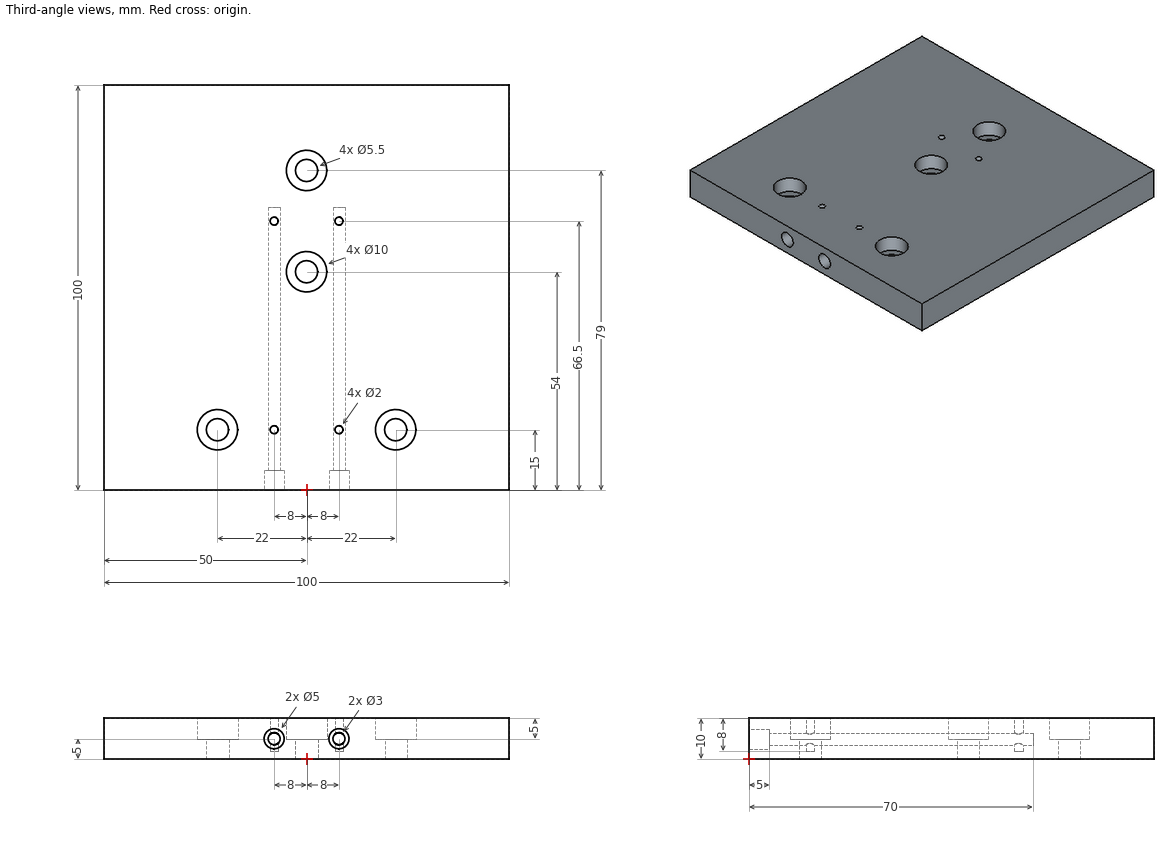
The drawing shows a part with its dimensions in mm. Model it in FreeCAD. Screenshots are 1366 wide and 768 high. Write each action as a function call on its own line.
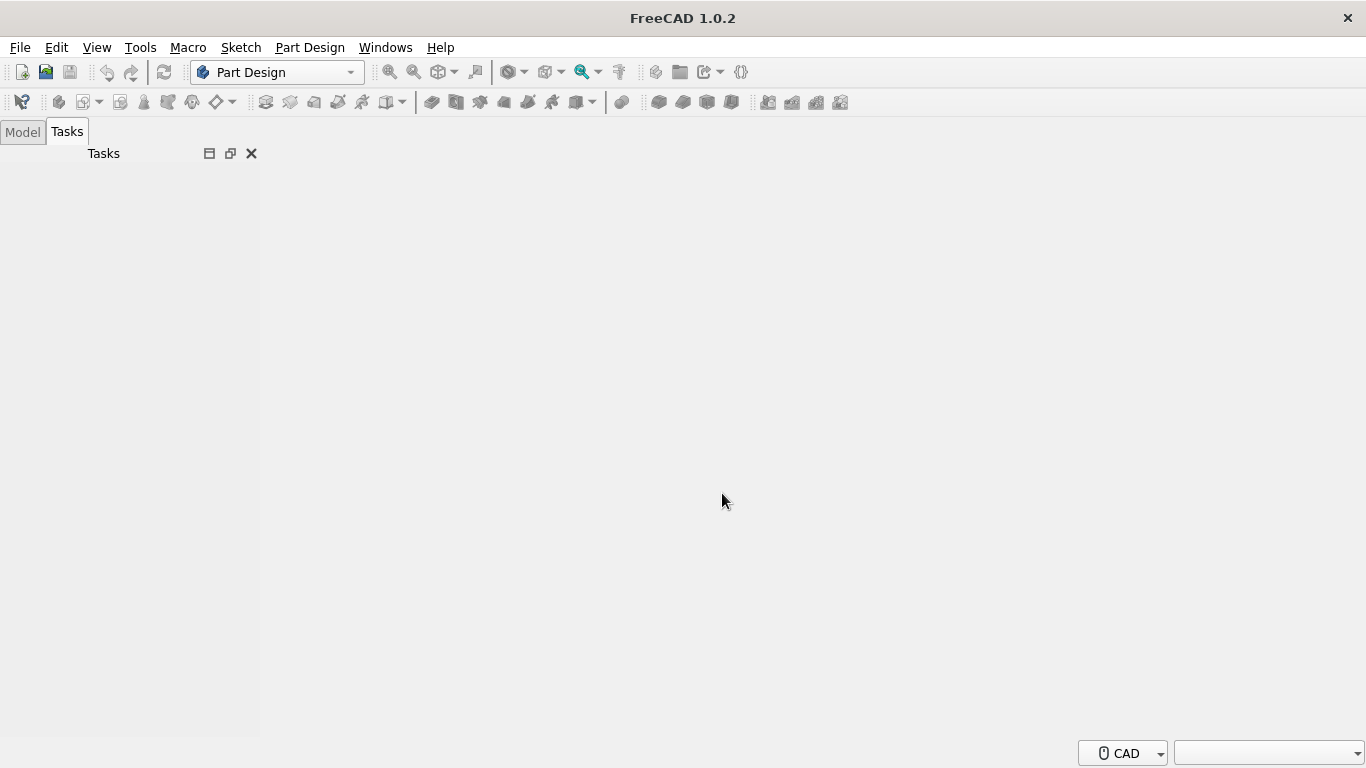
click(22, 72)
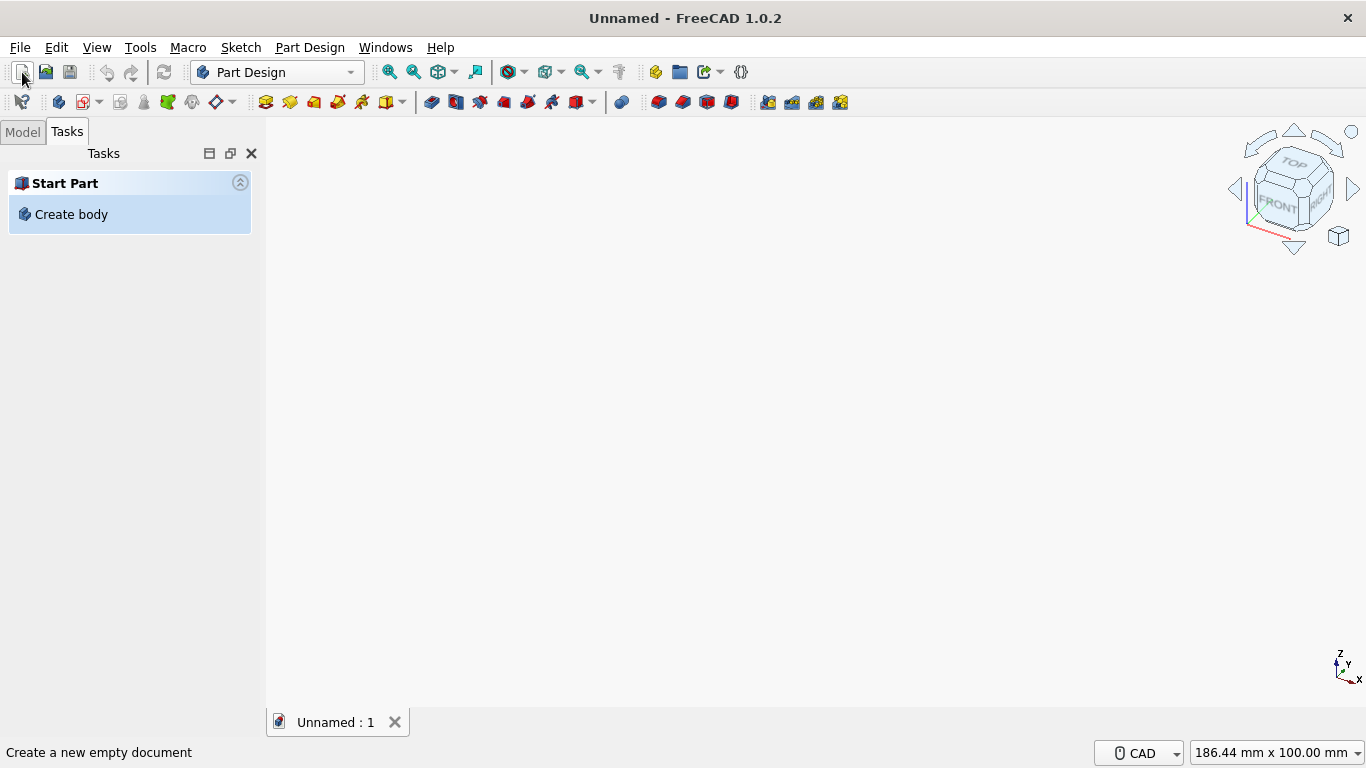
click(84, 102)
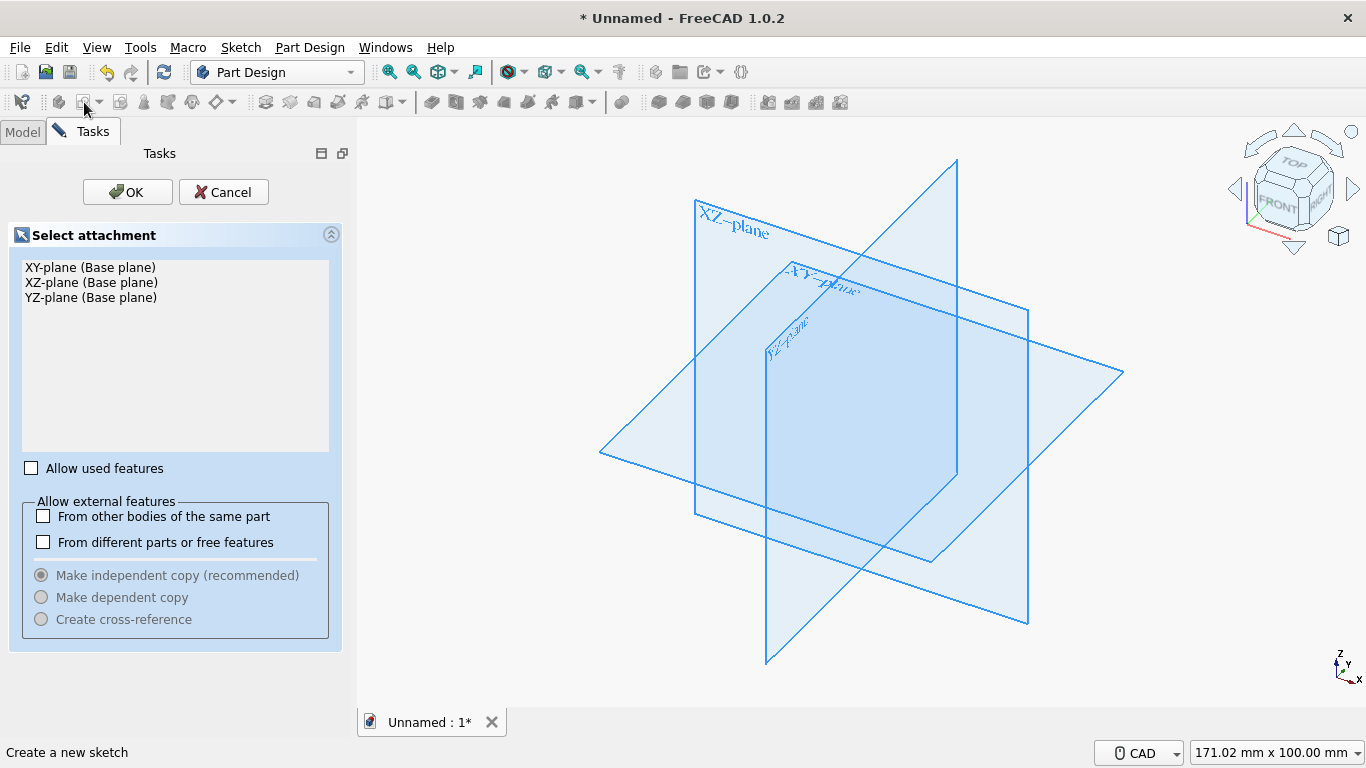
click(82, 268)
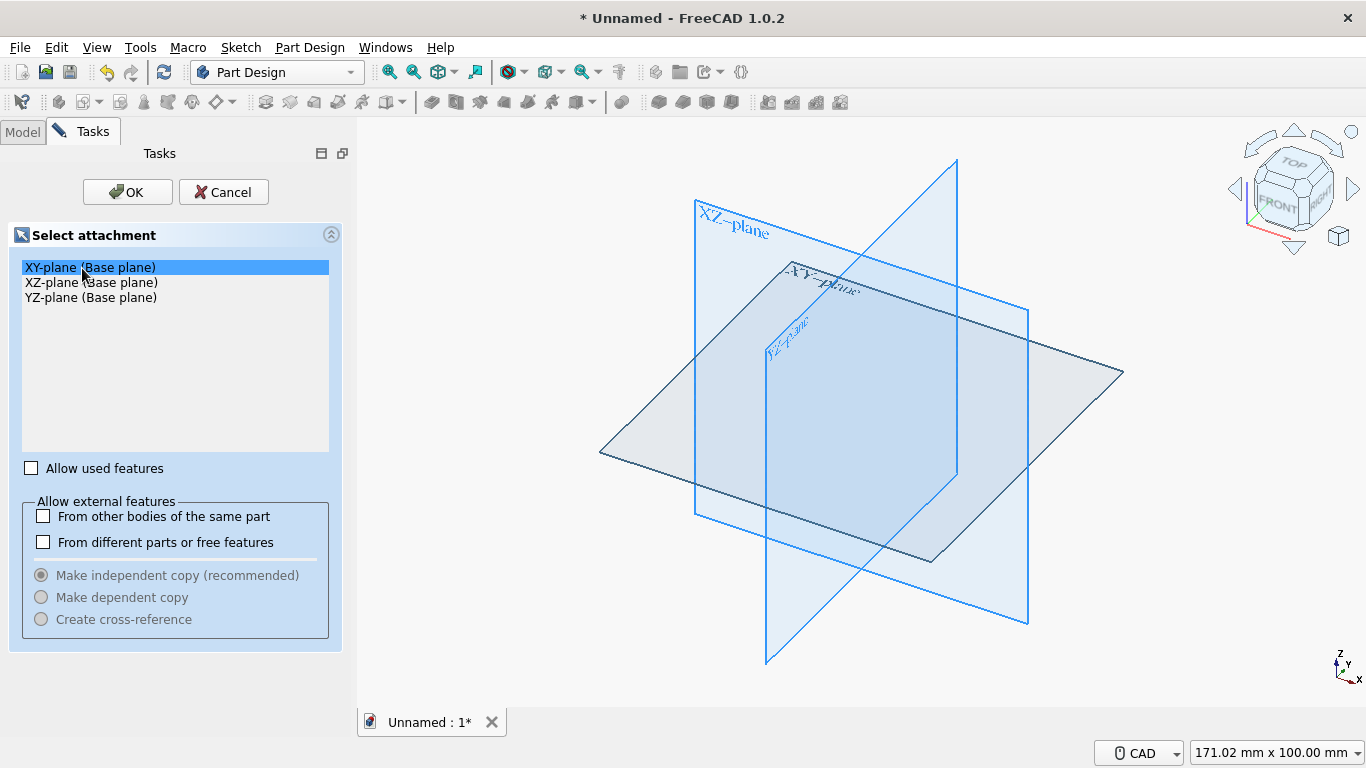
click(128, 192)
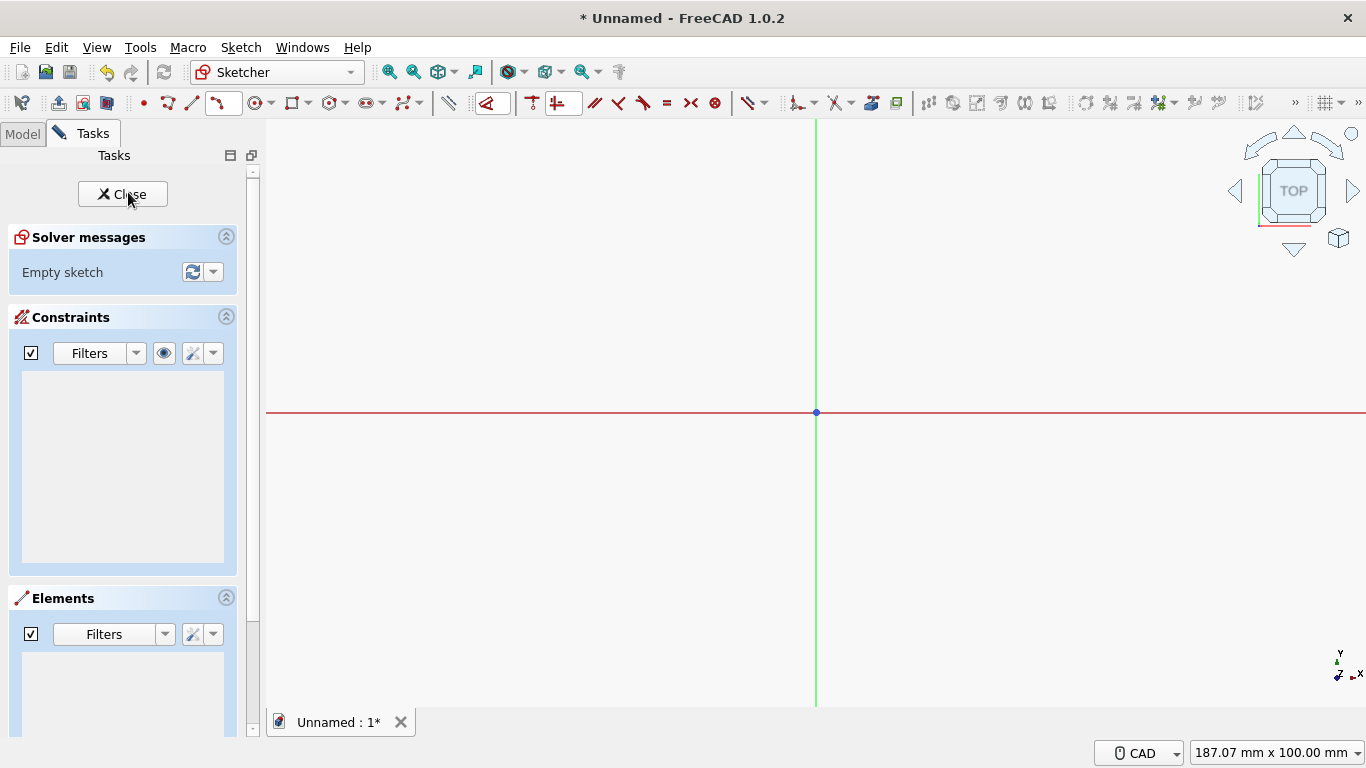
scroll(664, 679, down, 3)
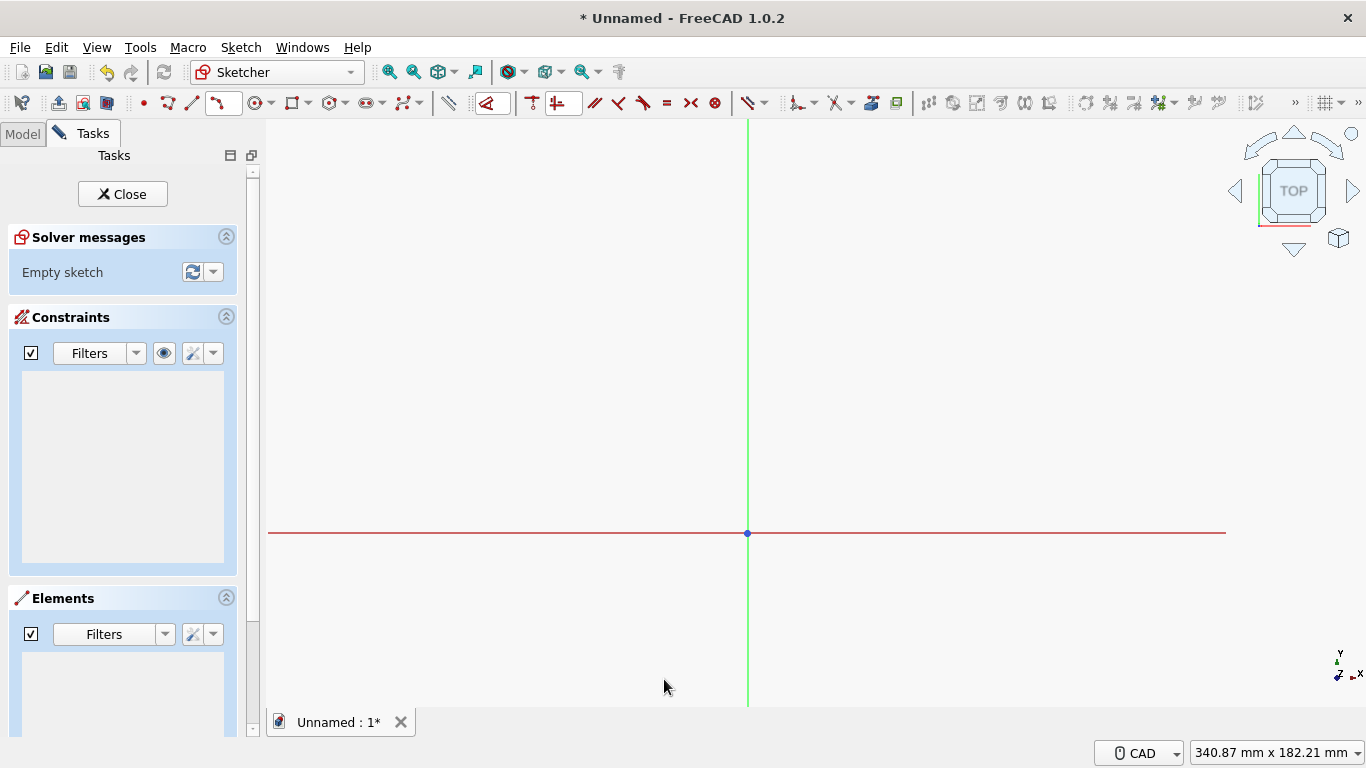
click(292, 104)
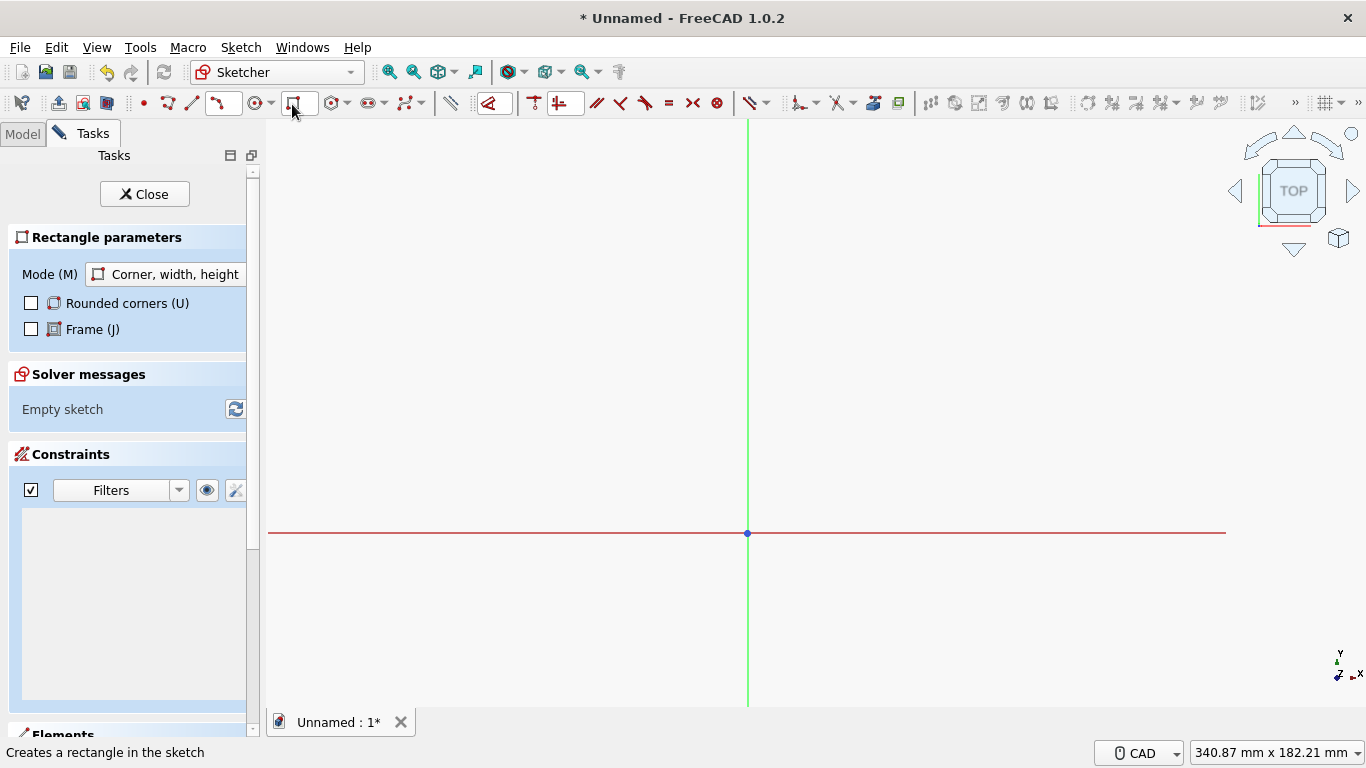
click(586, 211)
click(909, 533)
key(Escape)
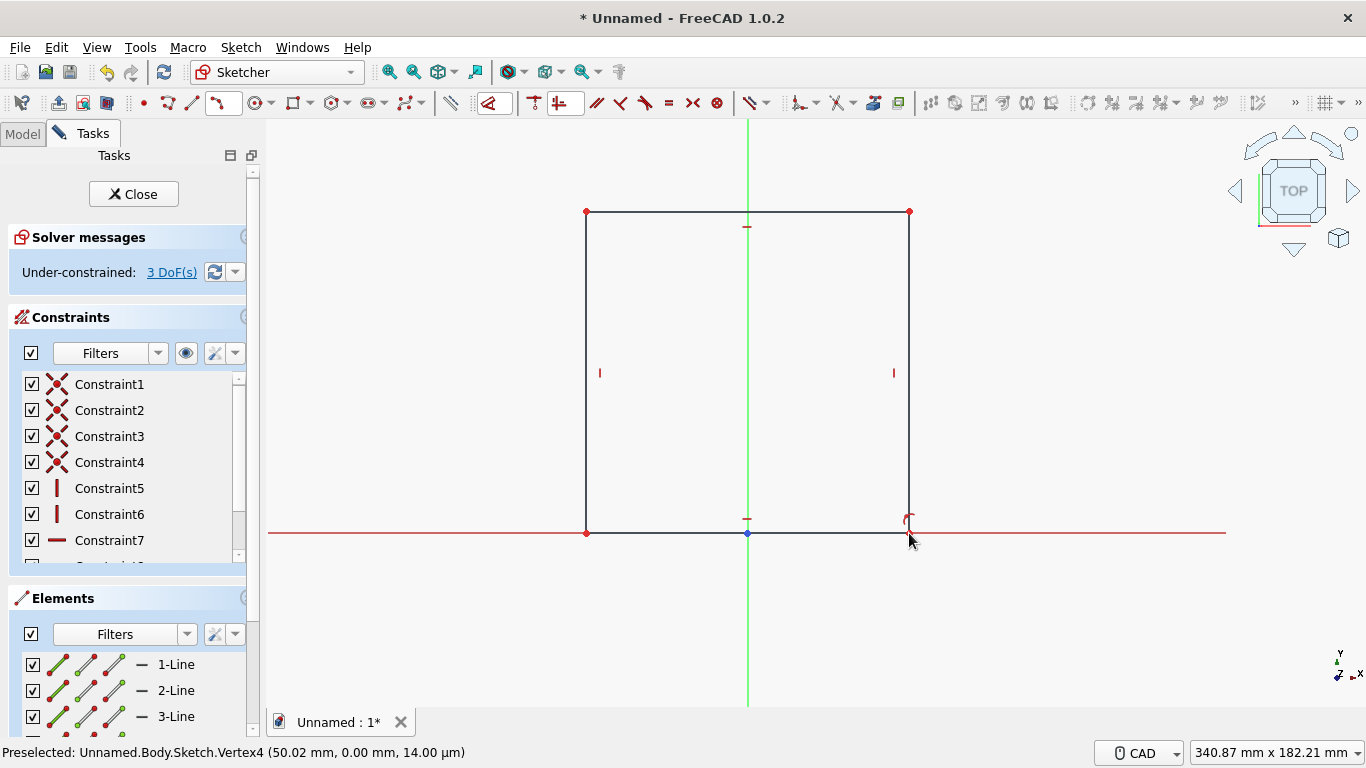
click(586, 308)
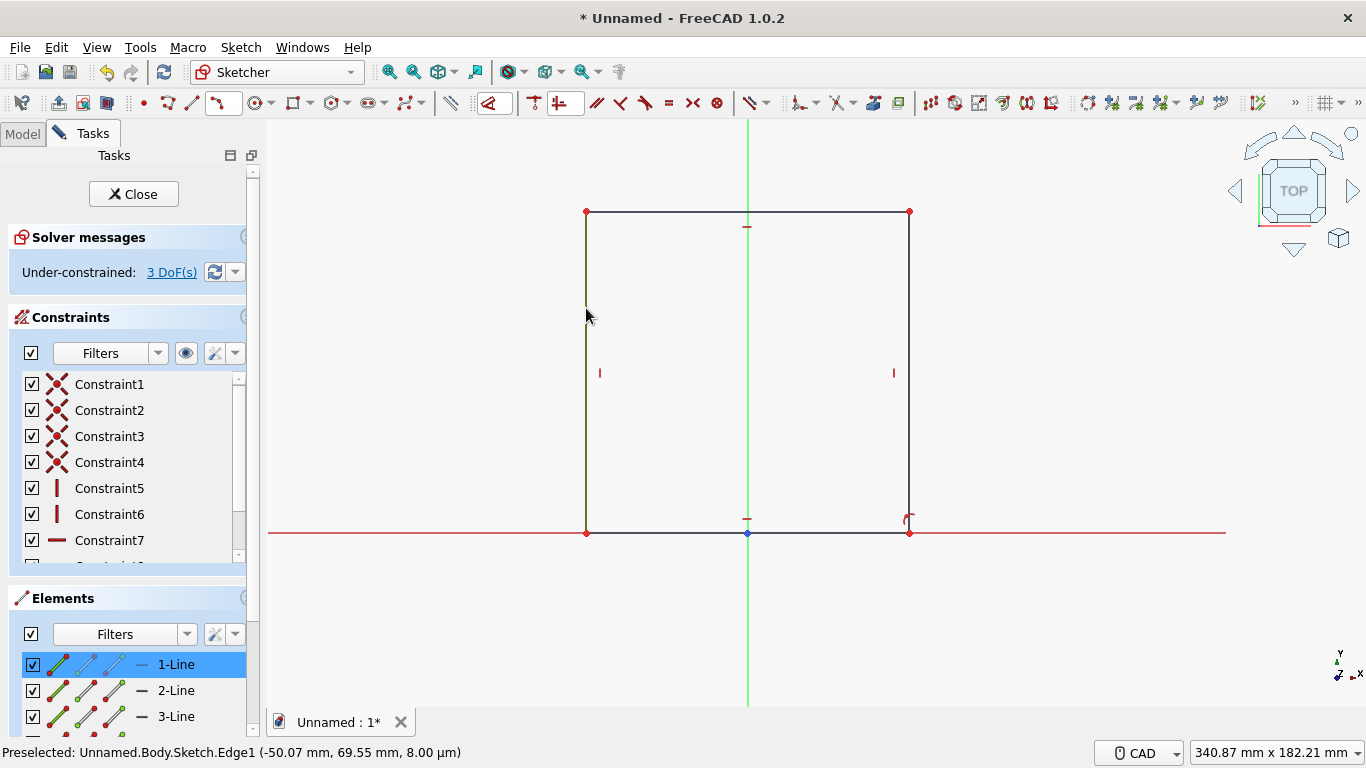
click(506, 104)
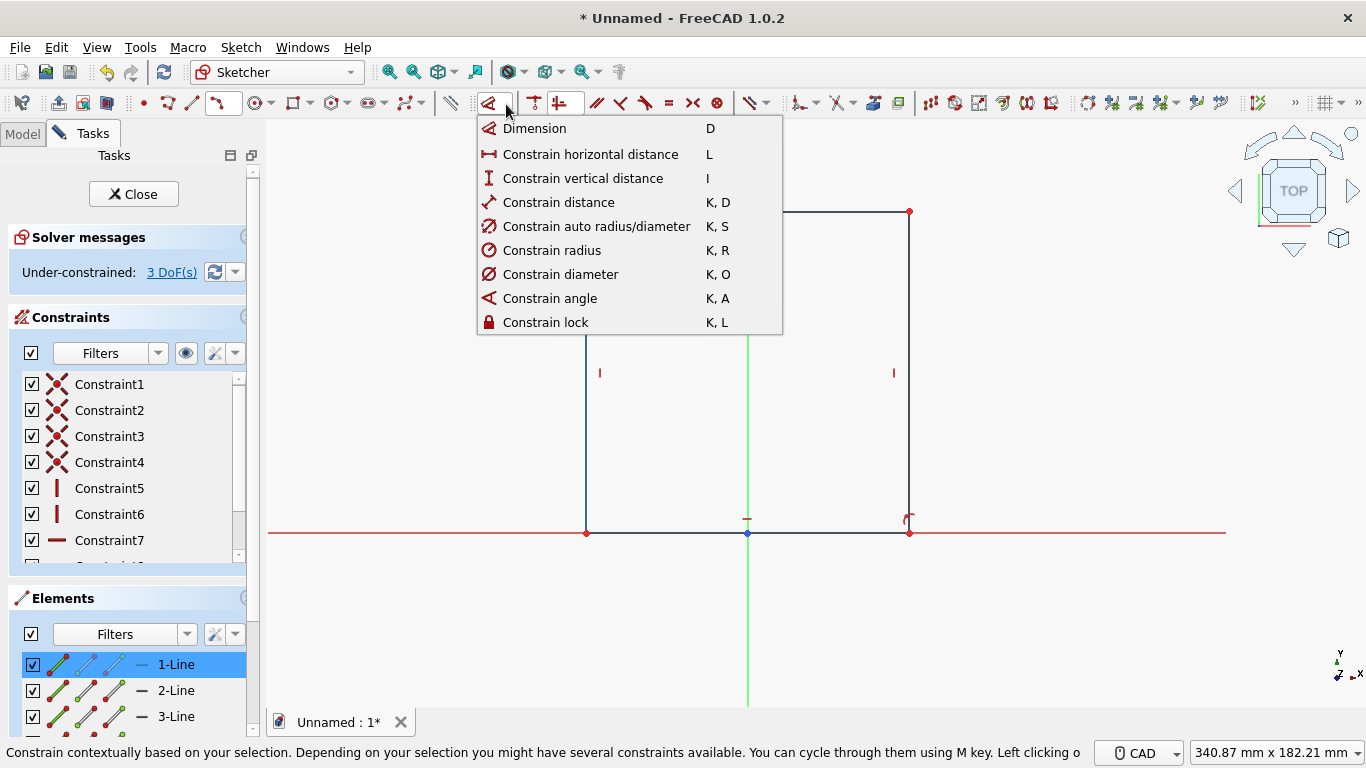
click(630, 178)